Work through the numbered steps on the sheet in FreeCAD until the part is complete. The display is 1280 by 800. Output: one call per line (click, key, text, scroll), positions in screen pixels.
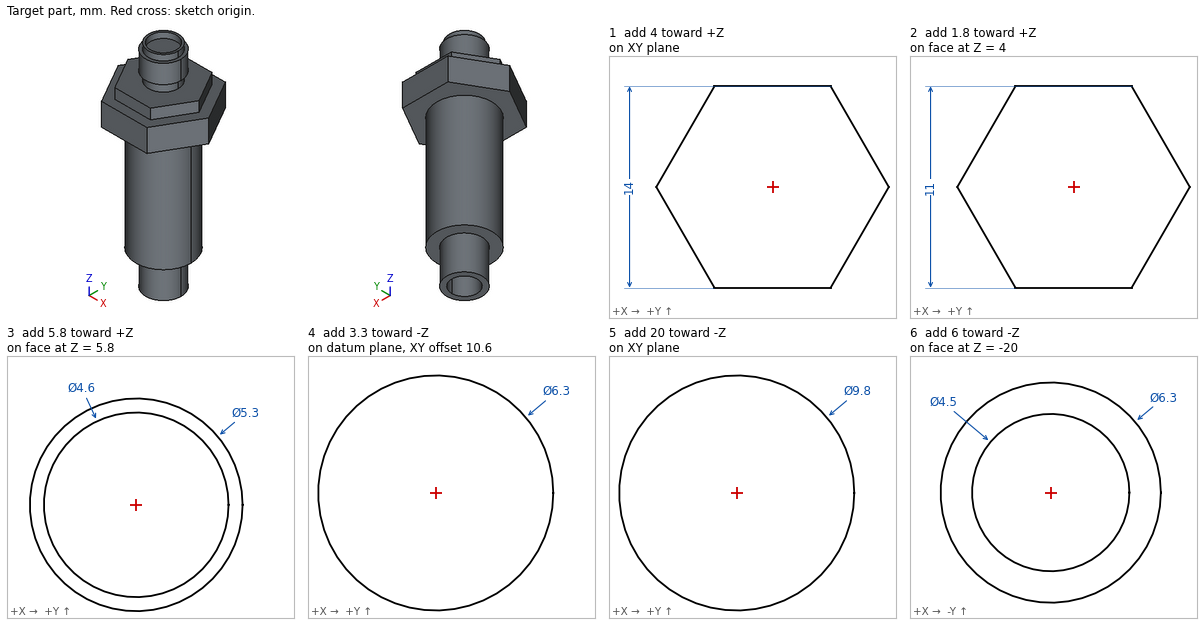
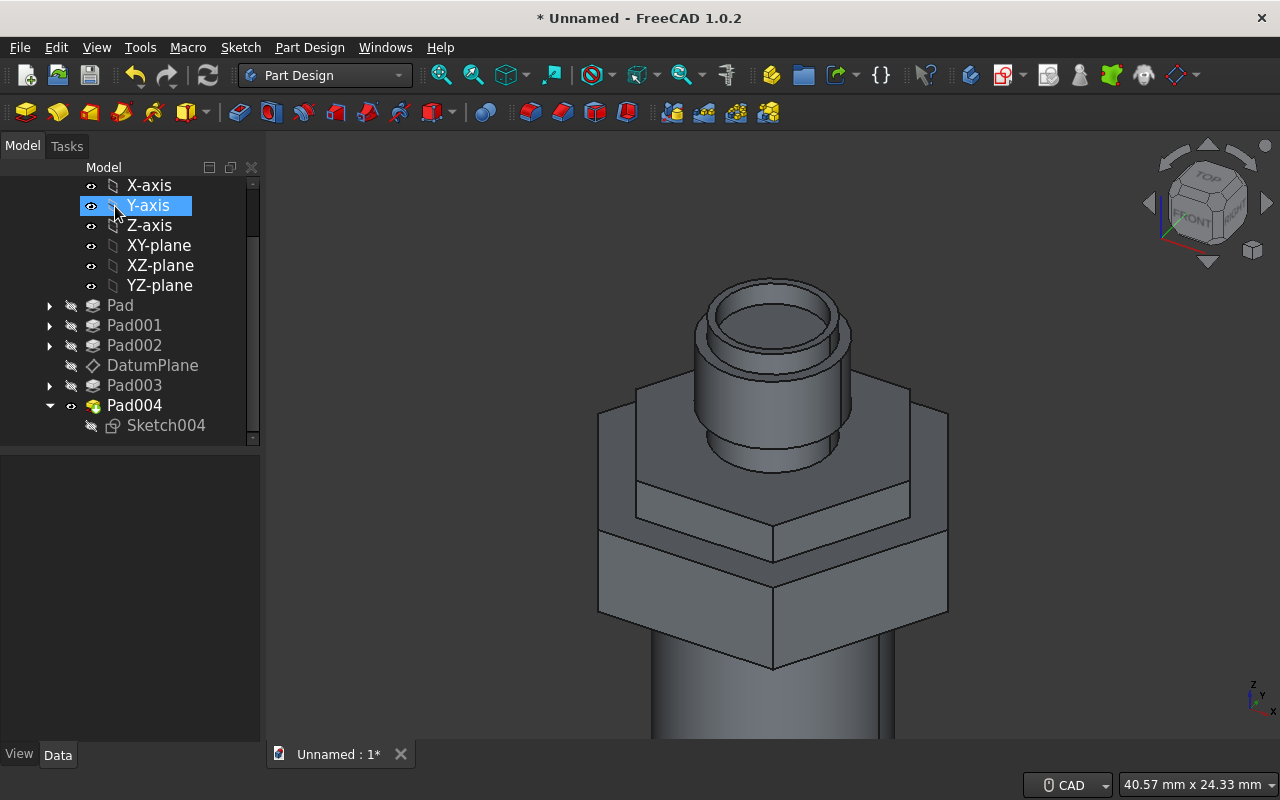
click(442, 76)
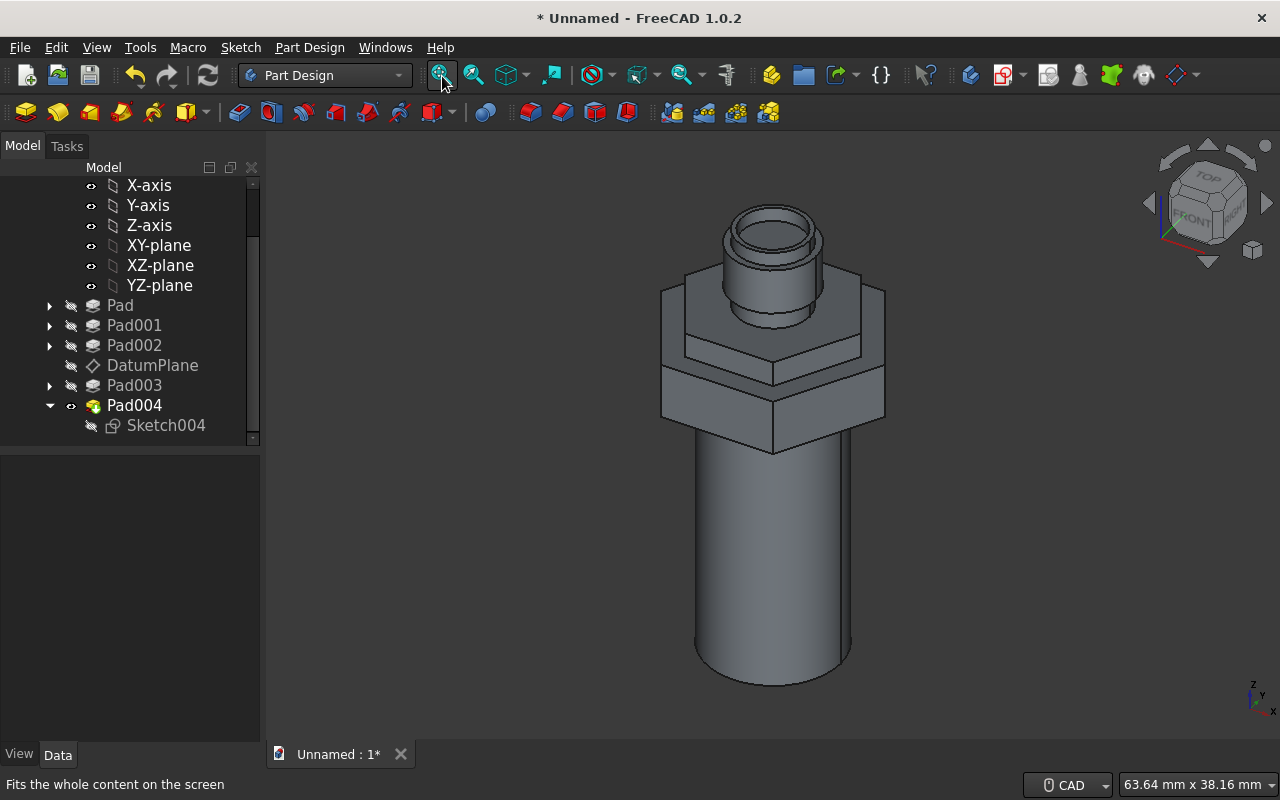
key(5)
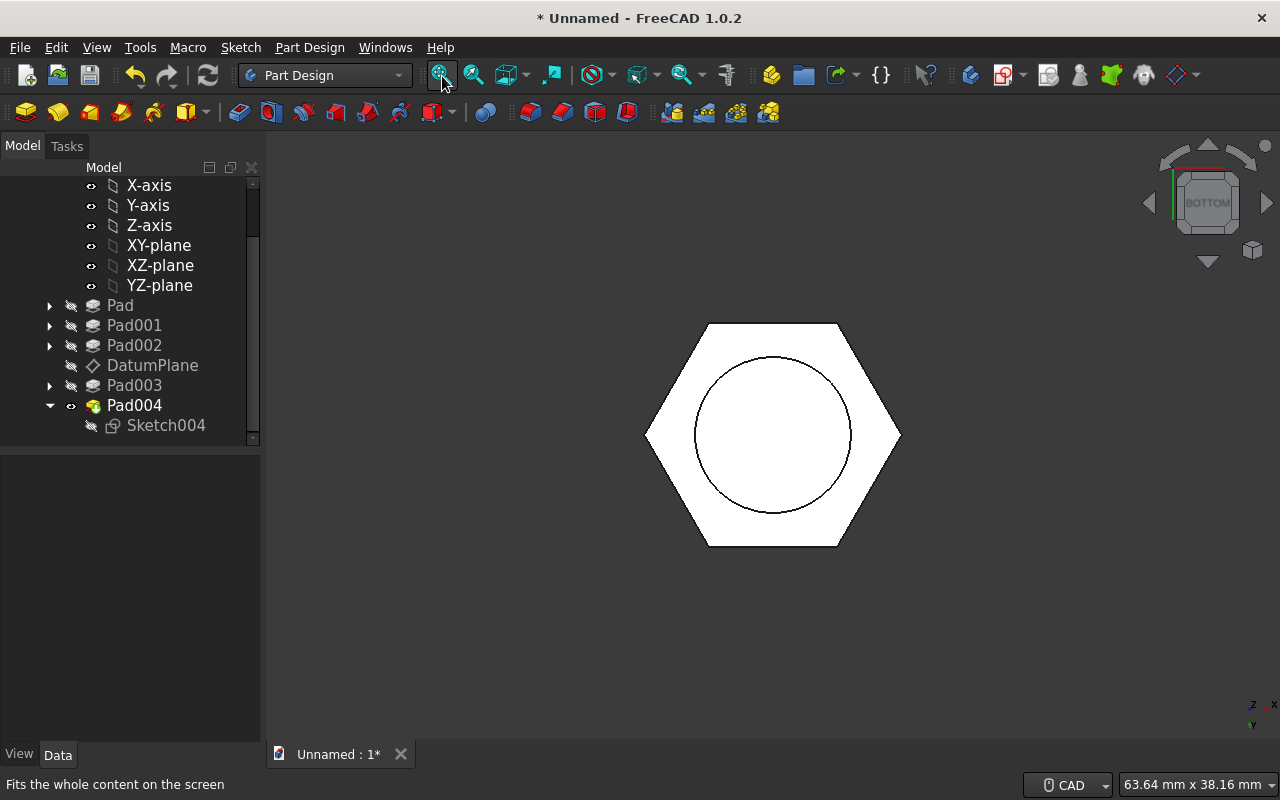
click(442, 76)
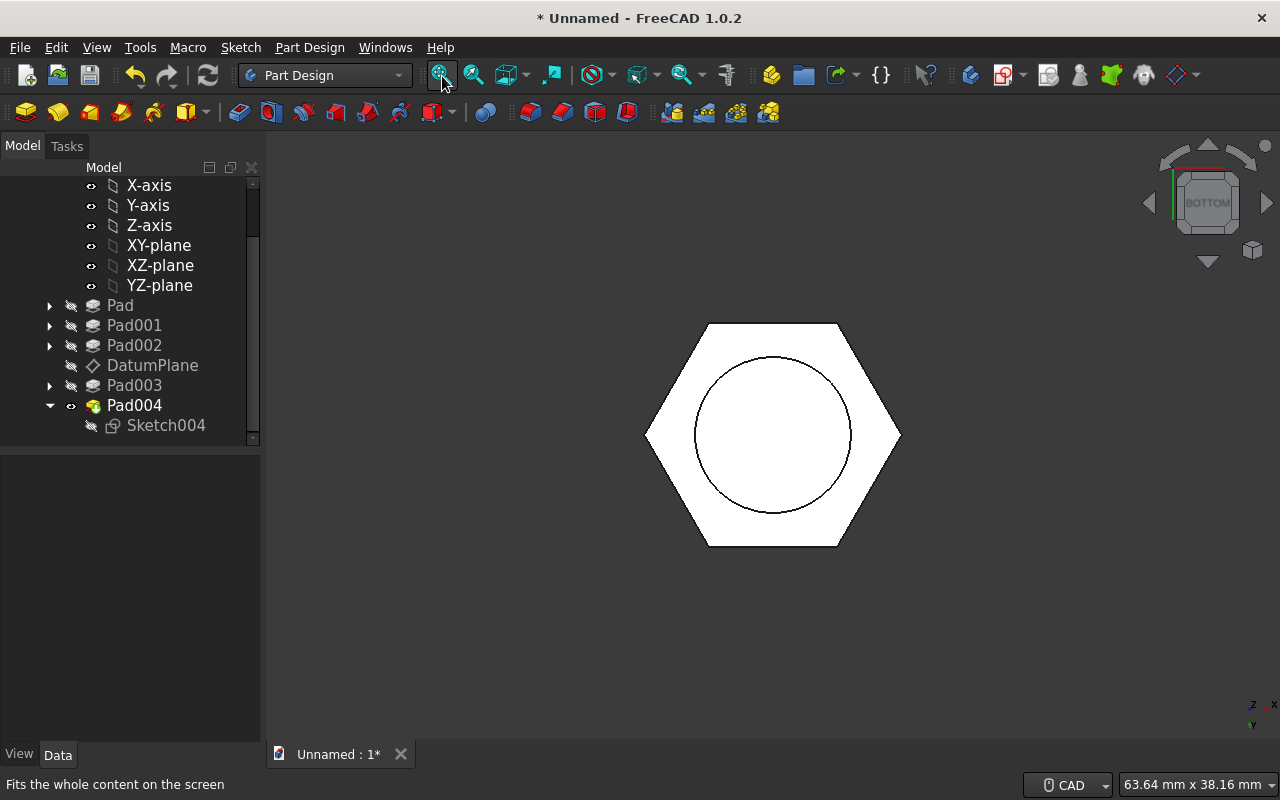
click(773, 434)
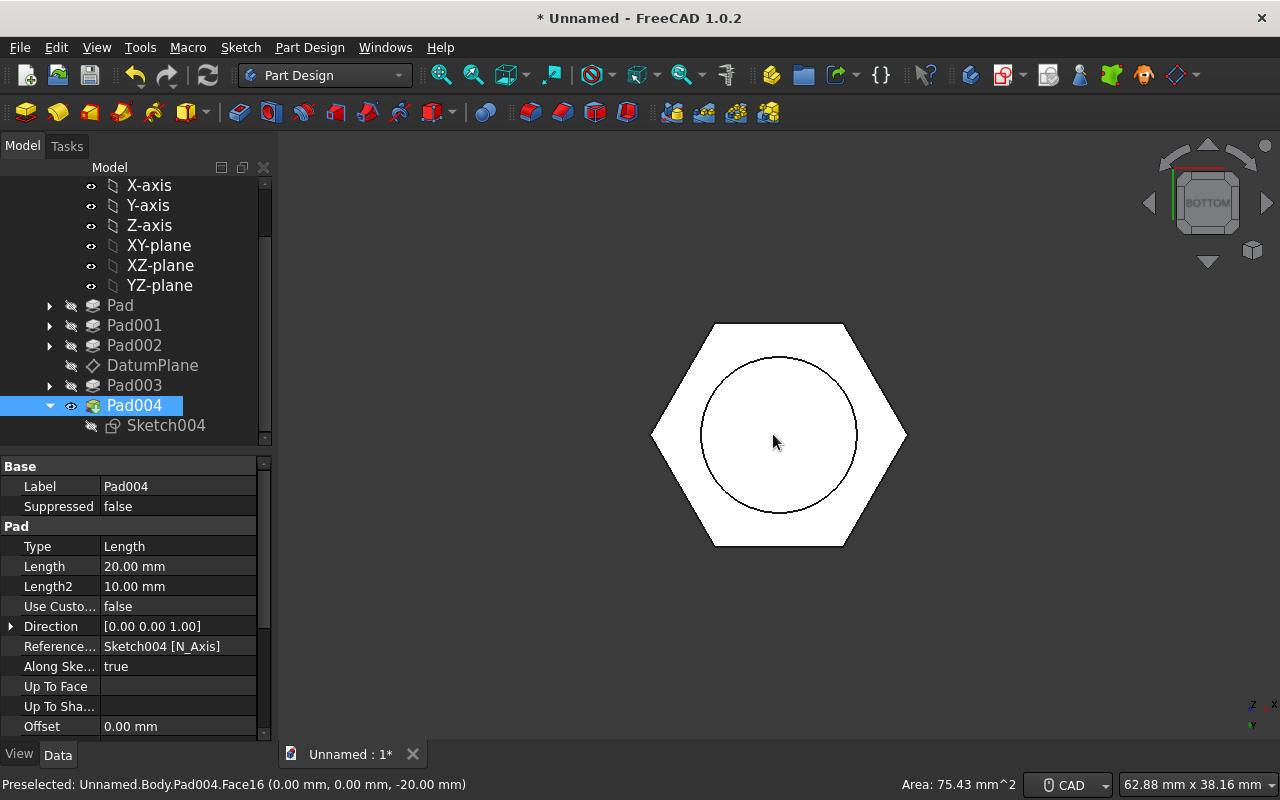
click(1004, 76)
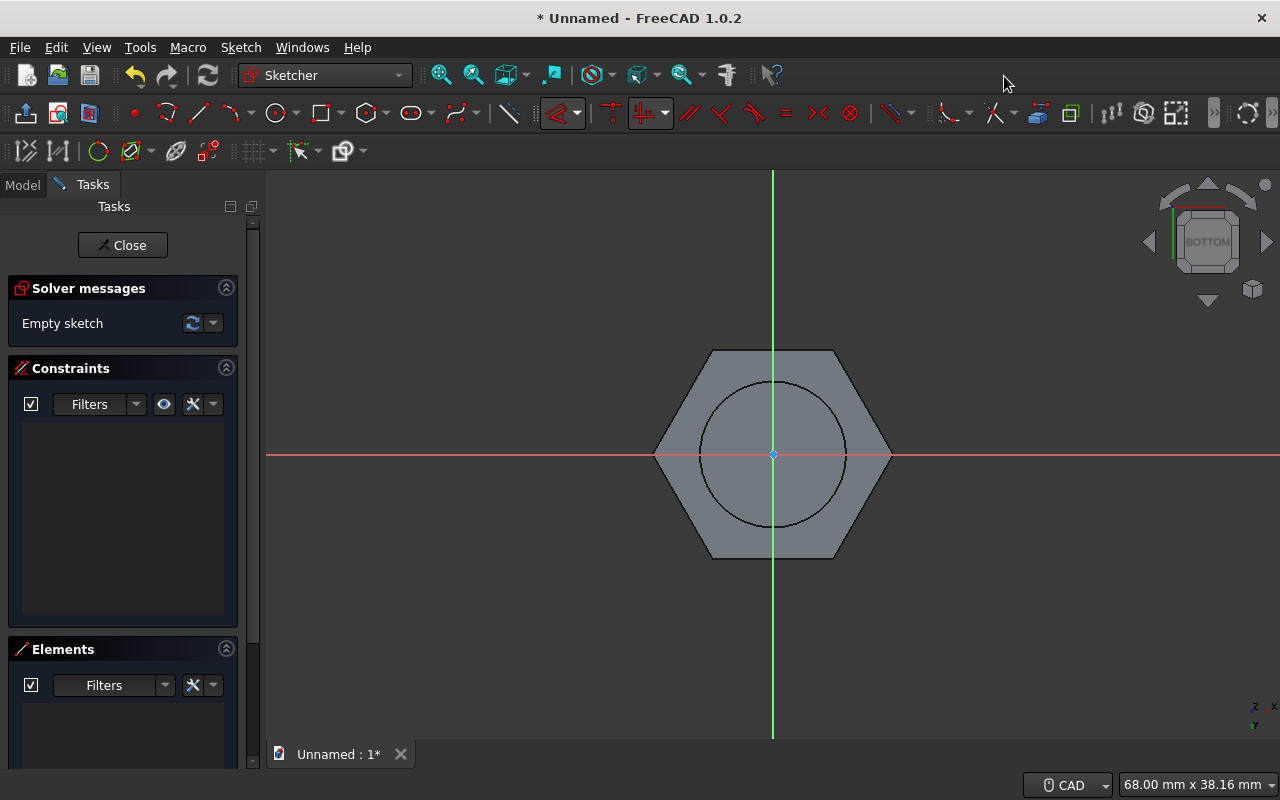
scroll(795, 454, up, 7)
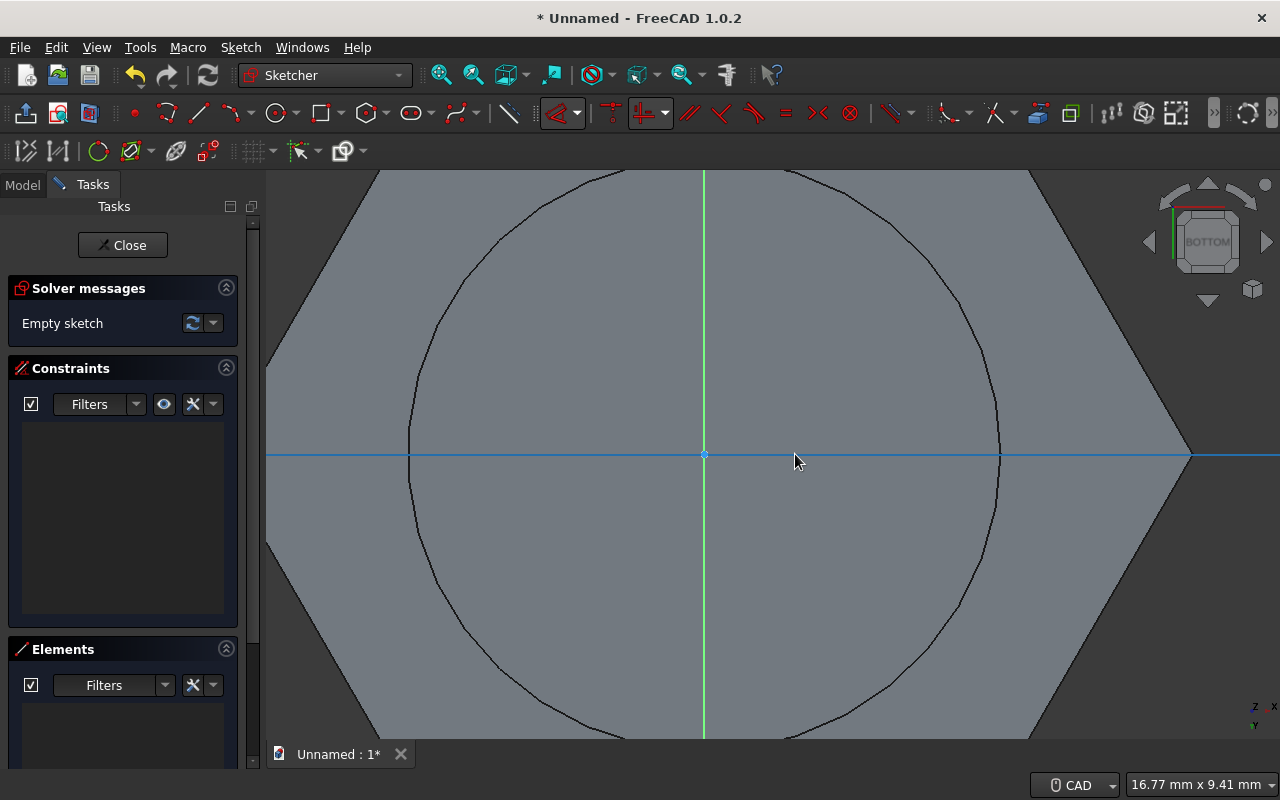
click(276, 114)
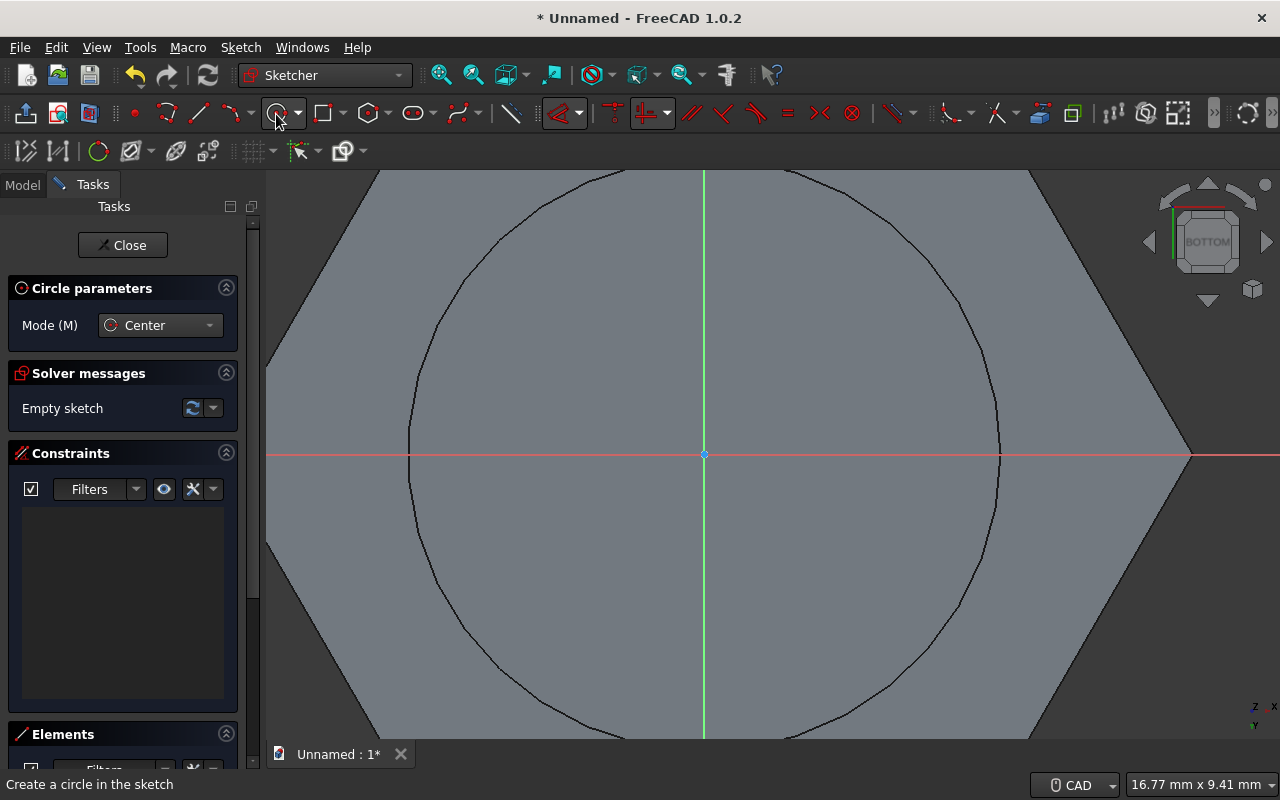
click(704, 454)
click(839, 320)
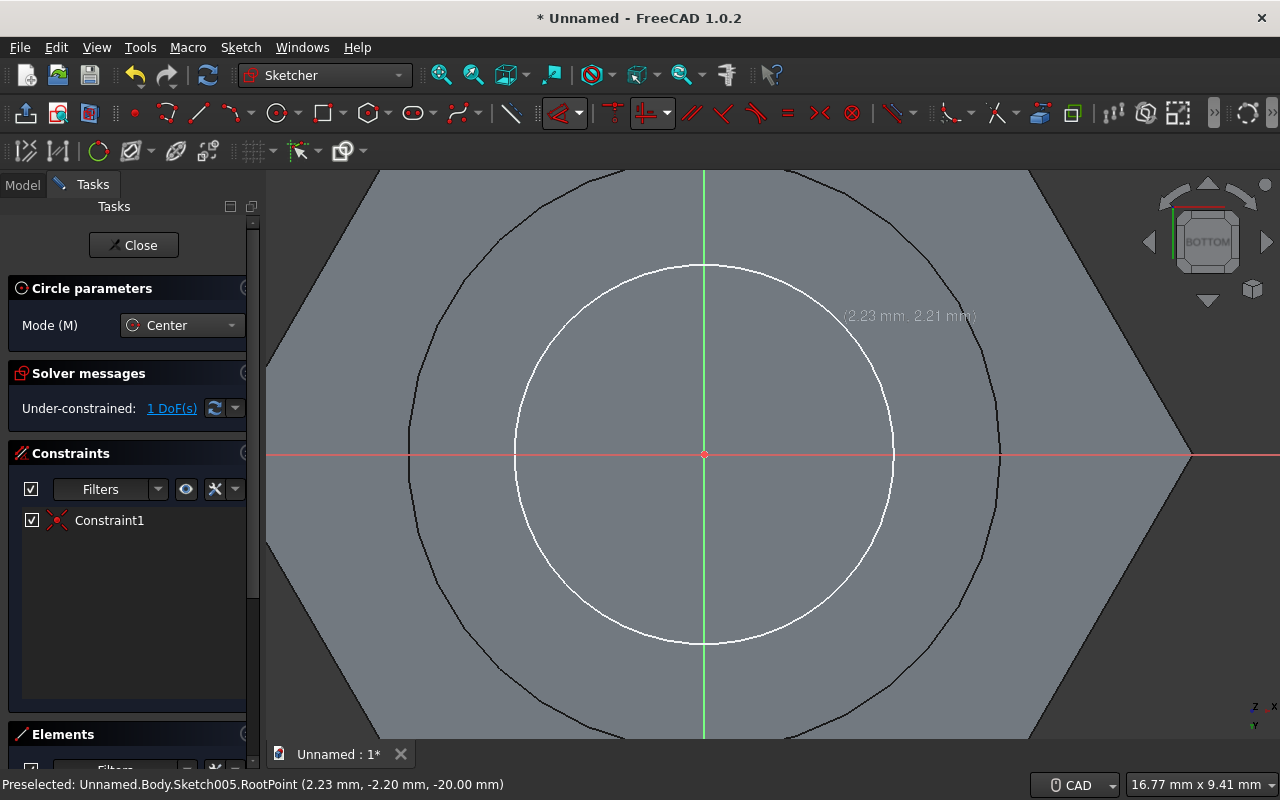
click(704, 454)
click(800, 358)
key(Escape)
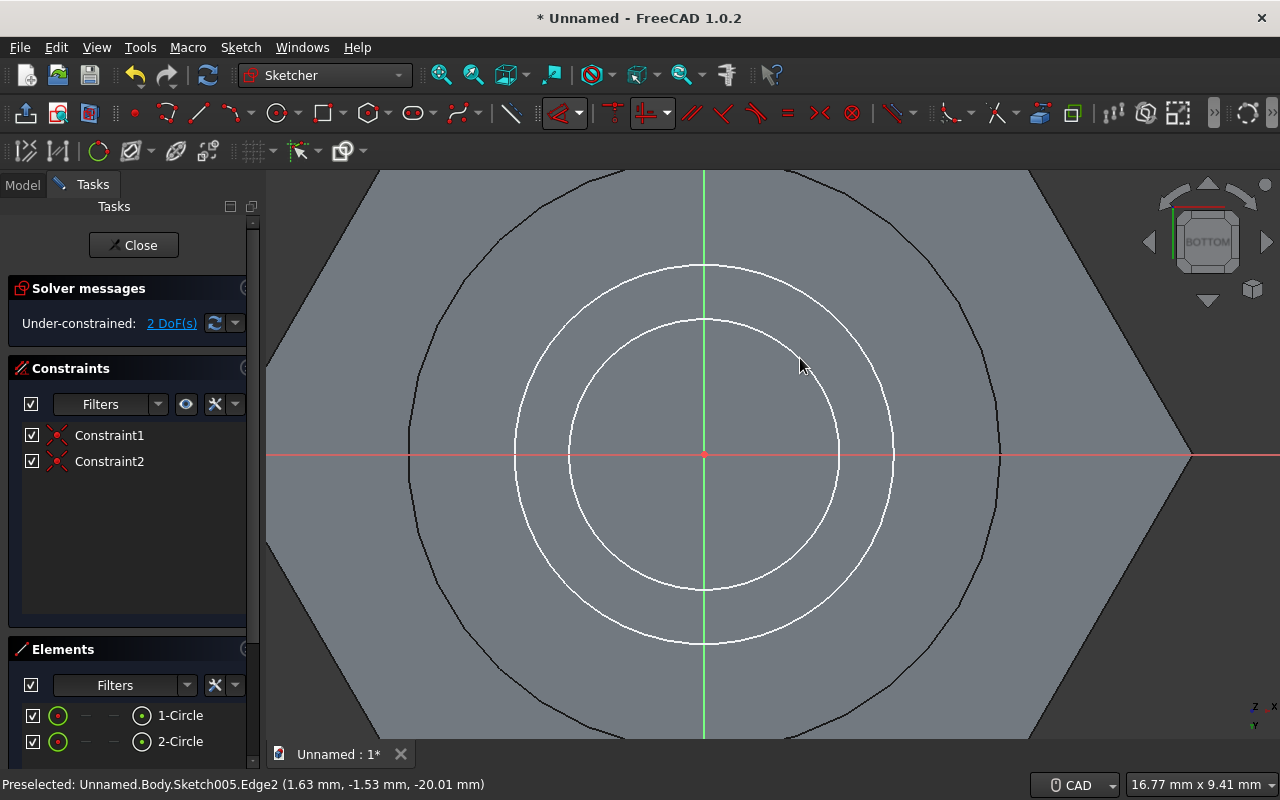
click(838, 320)